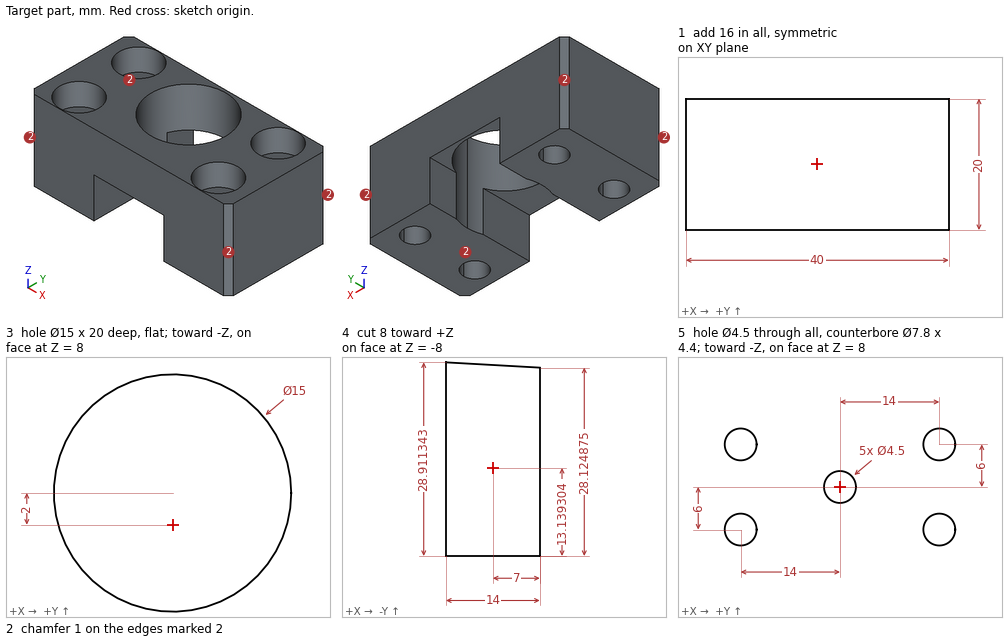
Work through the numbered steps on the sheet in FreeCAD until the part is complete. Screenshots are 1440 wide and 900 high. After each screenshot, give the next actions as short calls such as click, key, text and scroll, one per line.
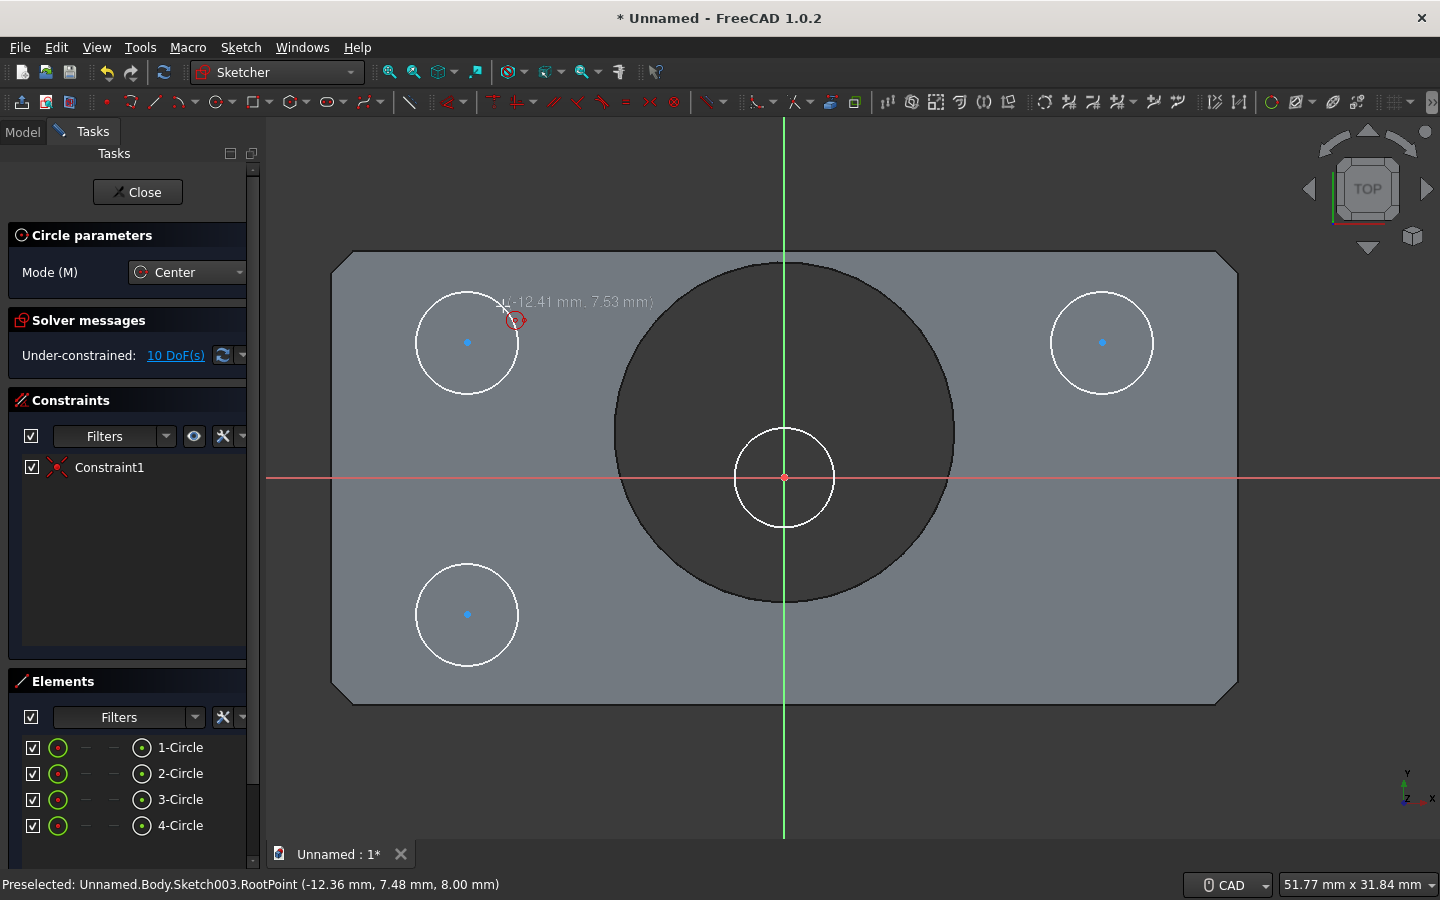
click(1102, 614)
click(1138, 578)
key(Escape)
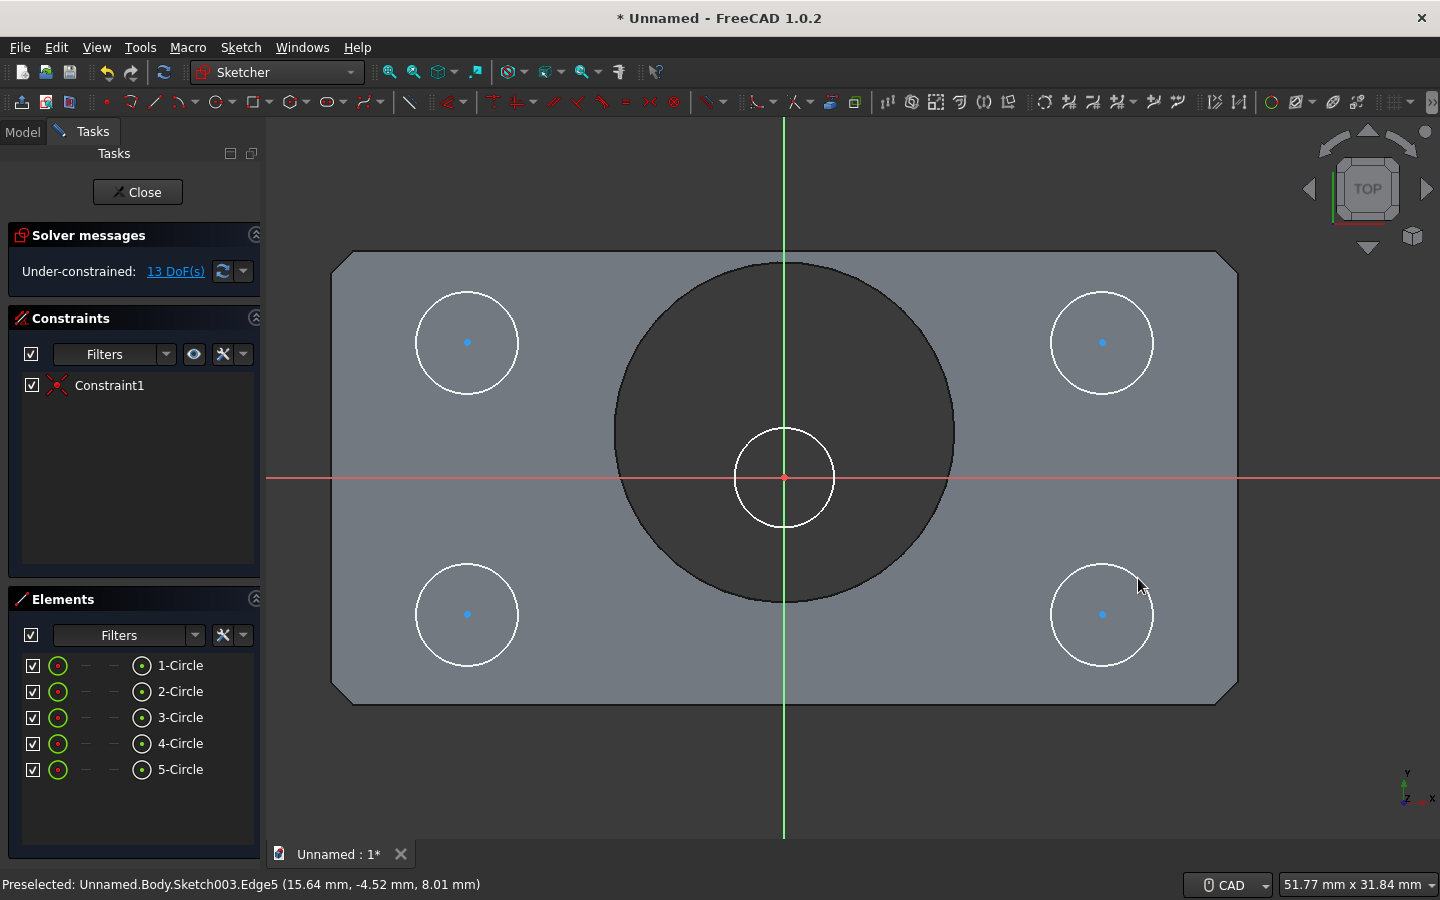
click(819, 442)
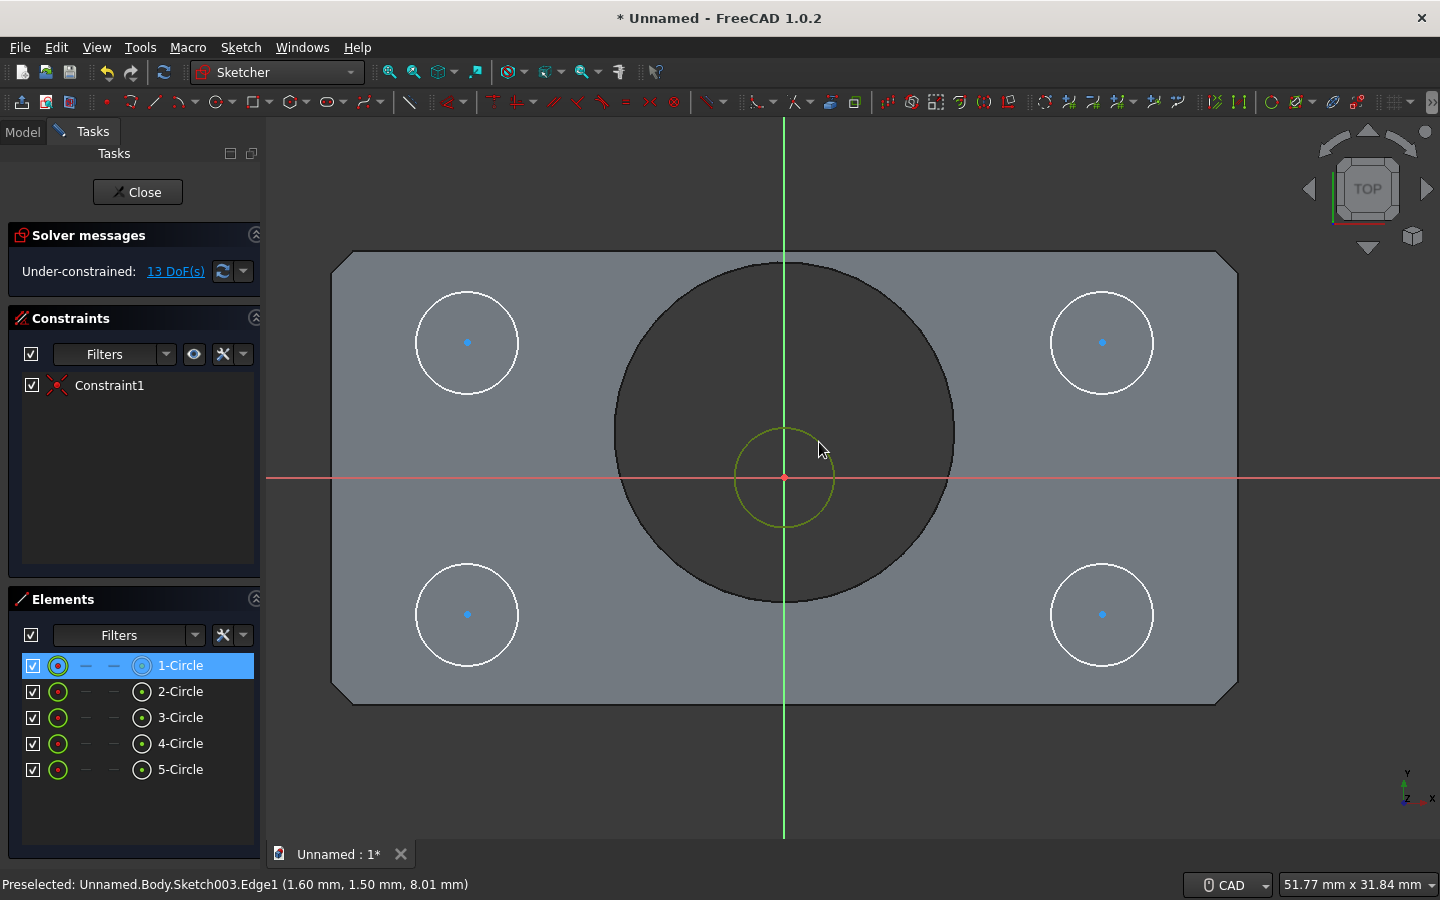
click(1138, 307)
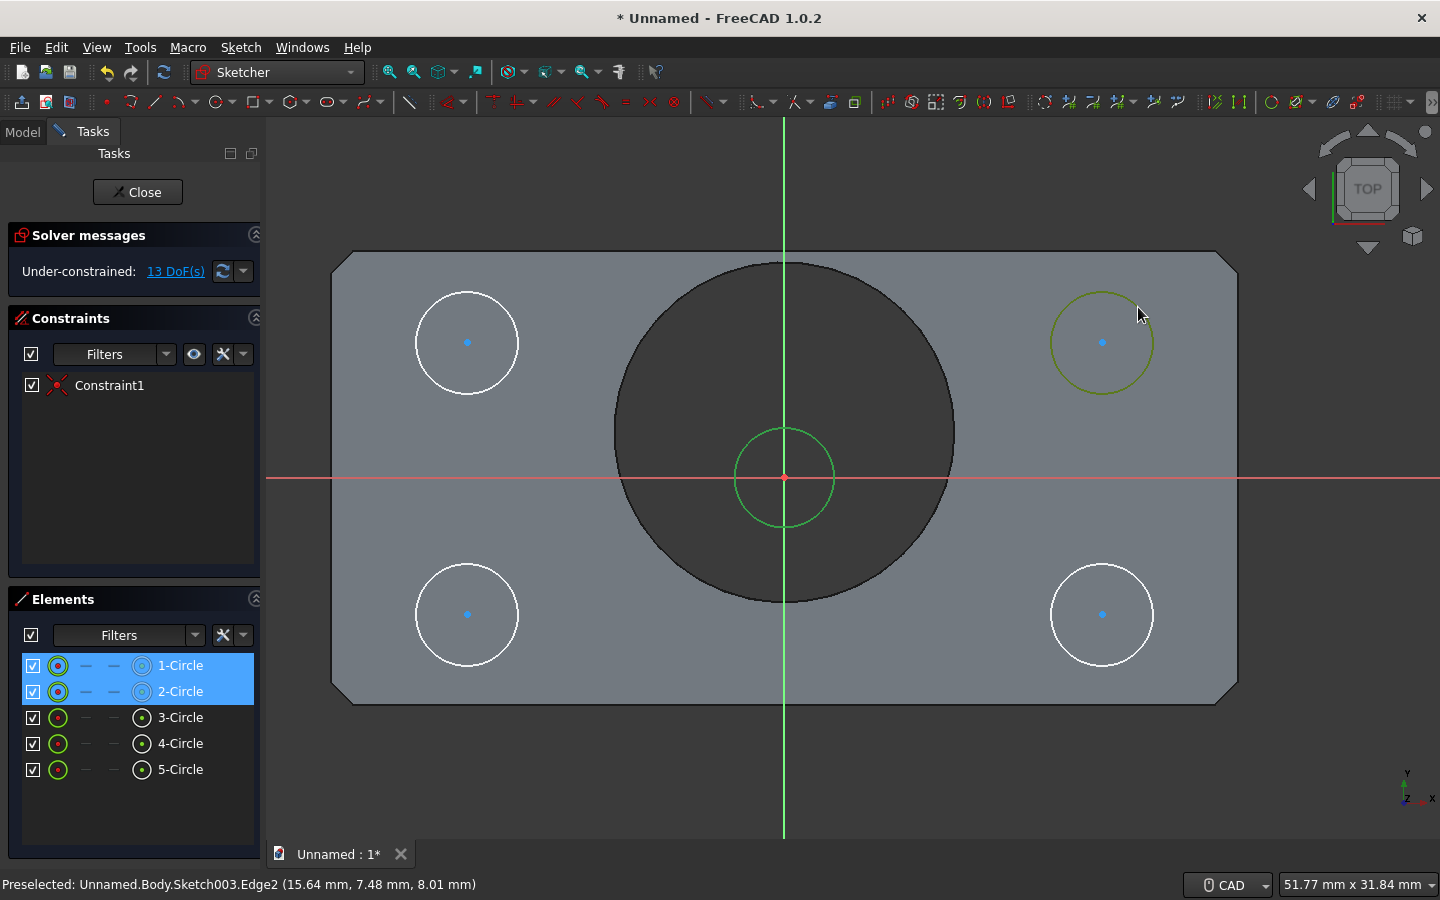
click(503, 579)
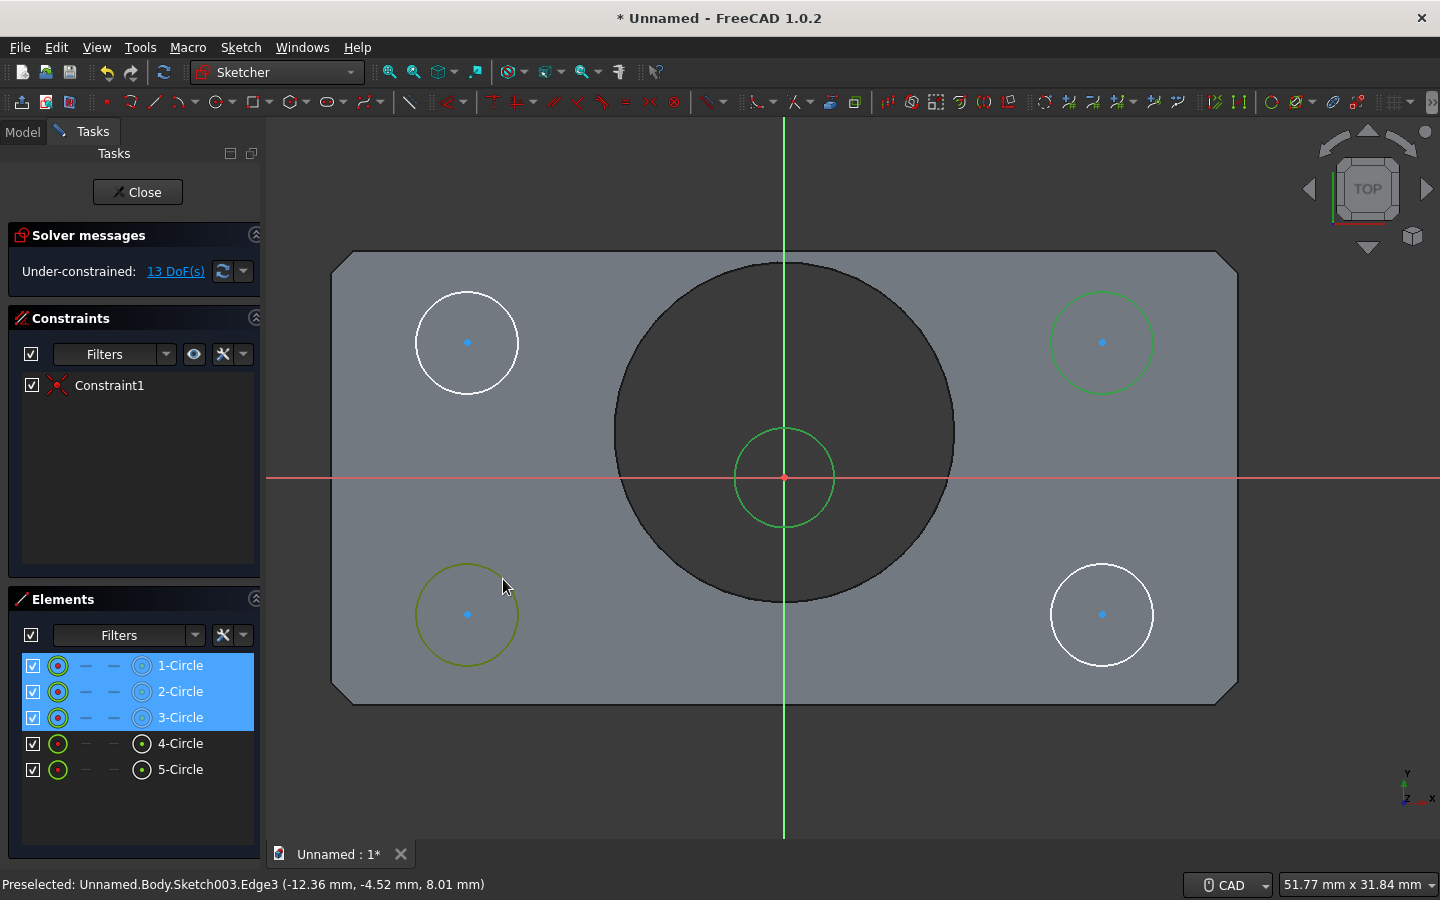
click(503, 307)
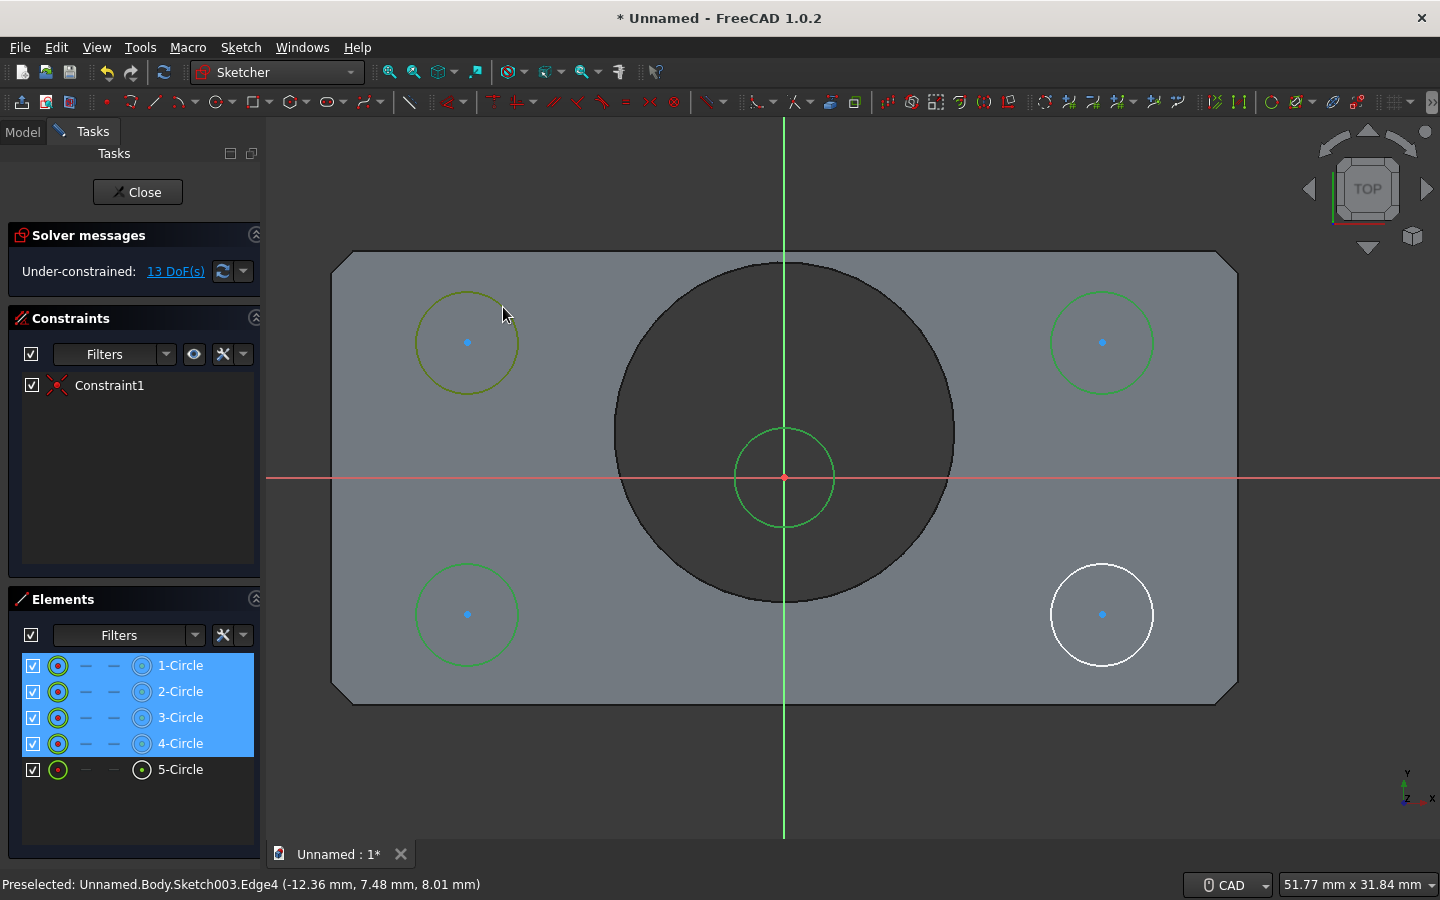
click(1138, 579)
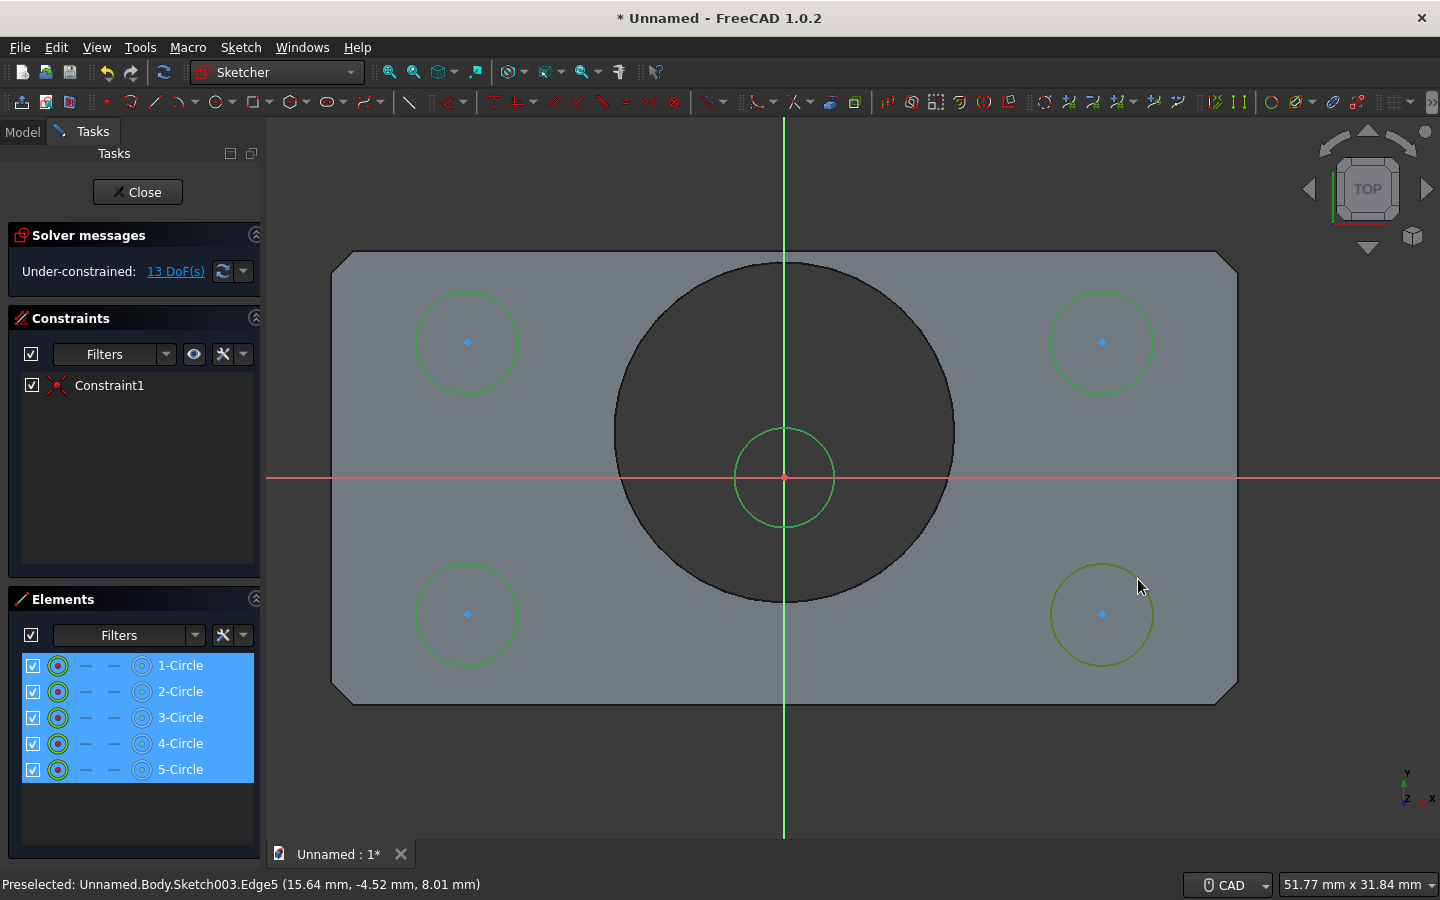
key(e)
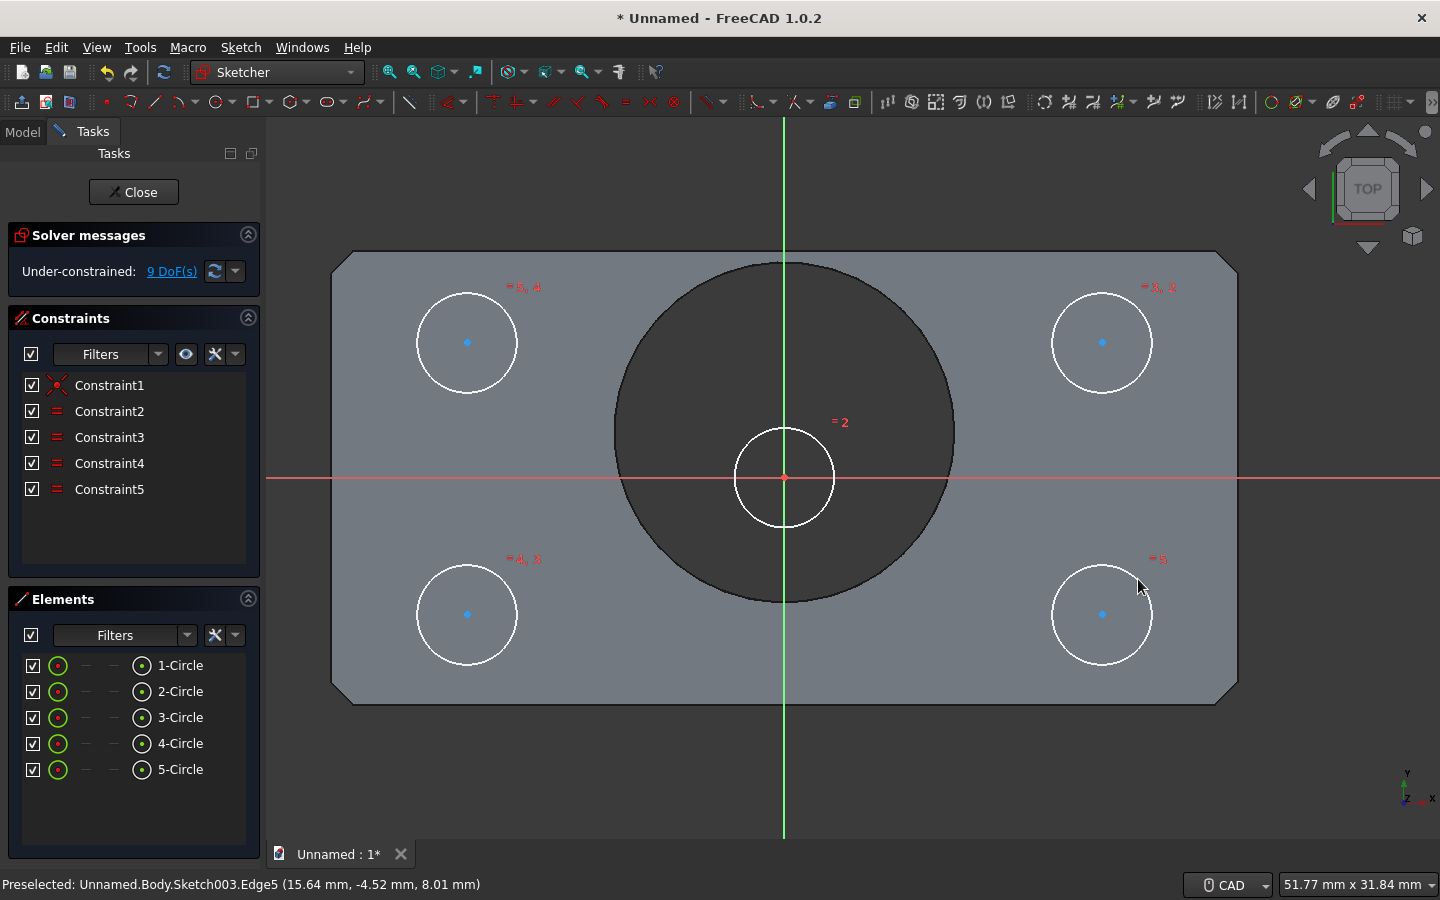
click(467, 615)